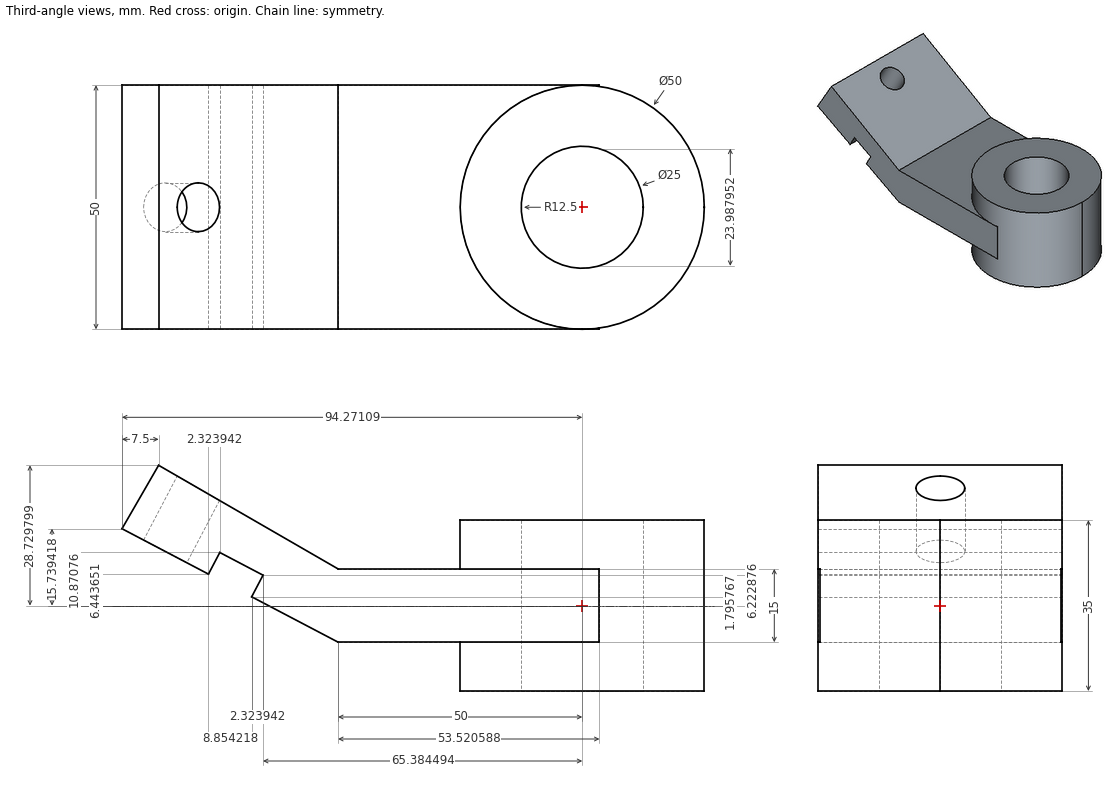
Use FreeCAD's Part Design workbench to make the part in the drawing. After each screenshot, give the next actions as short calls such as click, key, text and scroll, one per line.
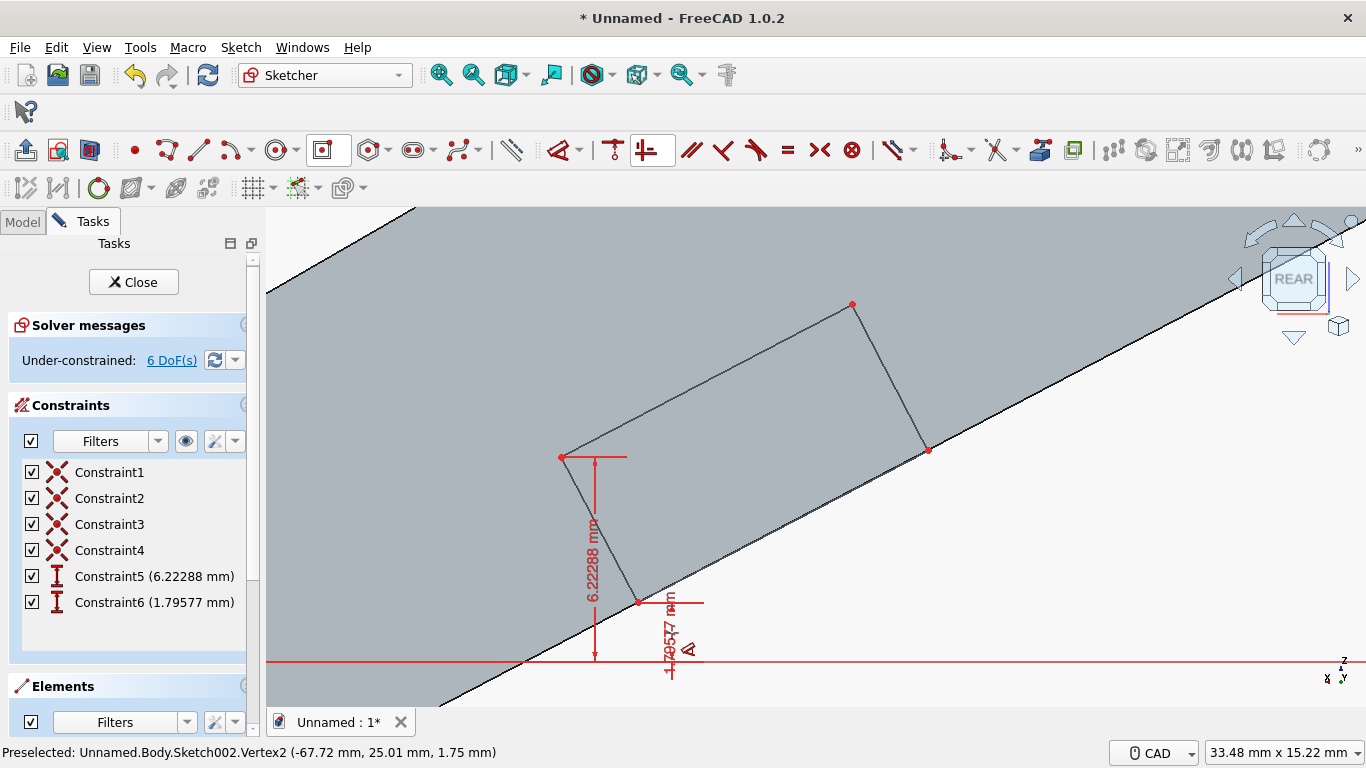
click(928, 451)
click(962, 556)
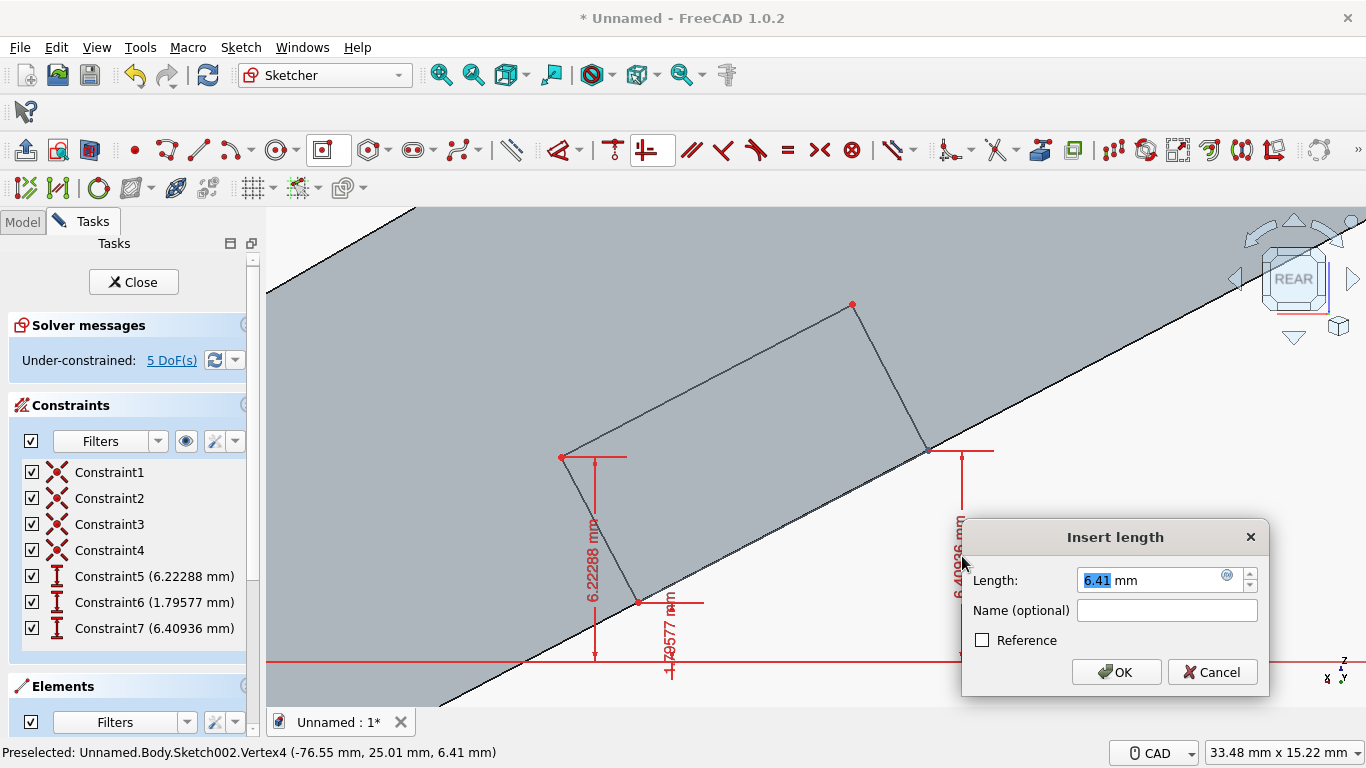
text(6.443651)
key(Return)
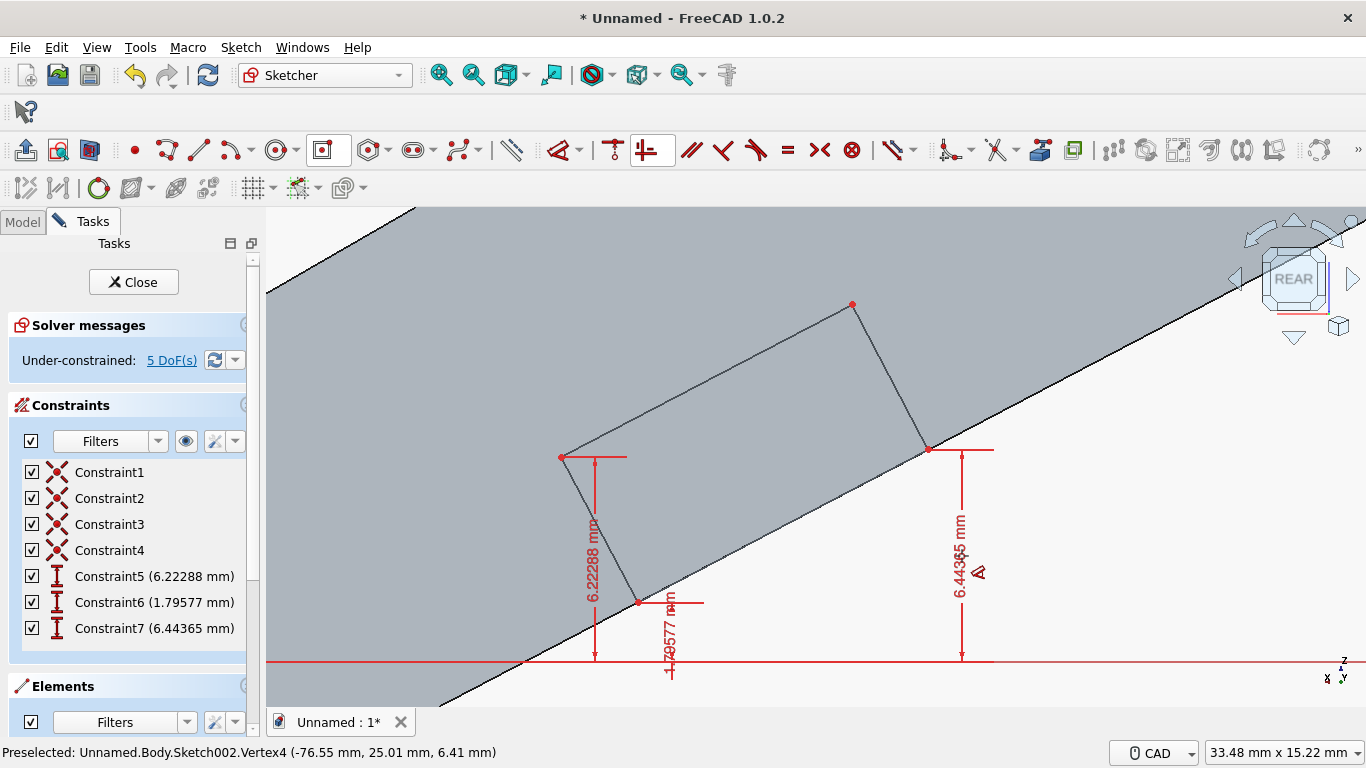
click(852, 305)
click(886, 401)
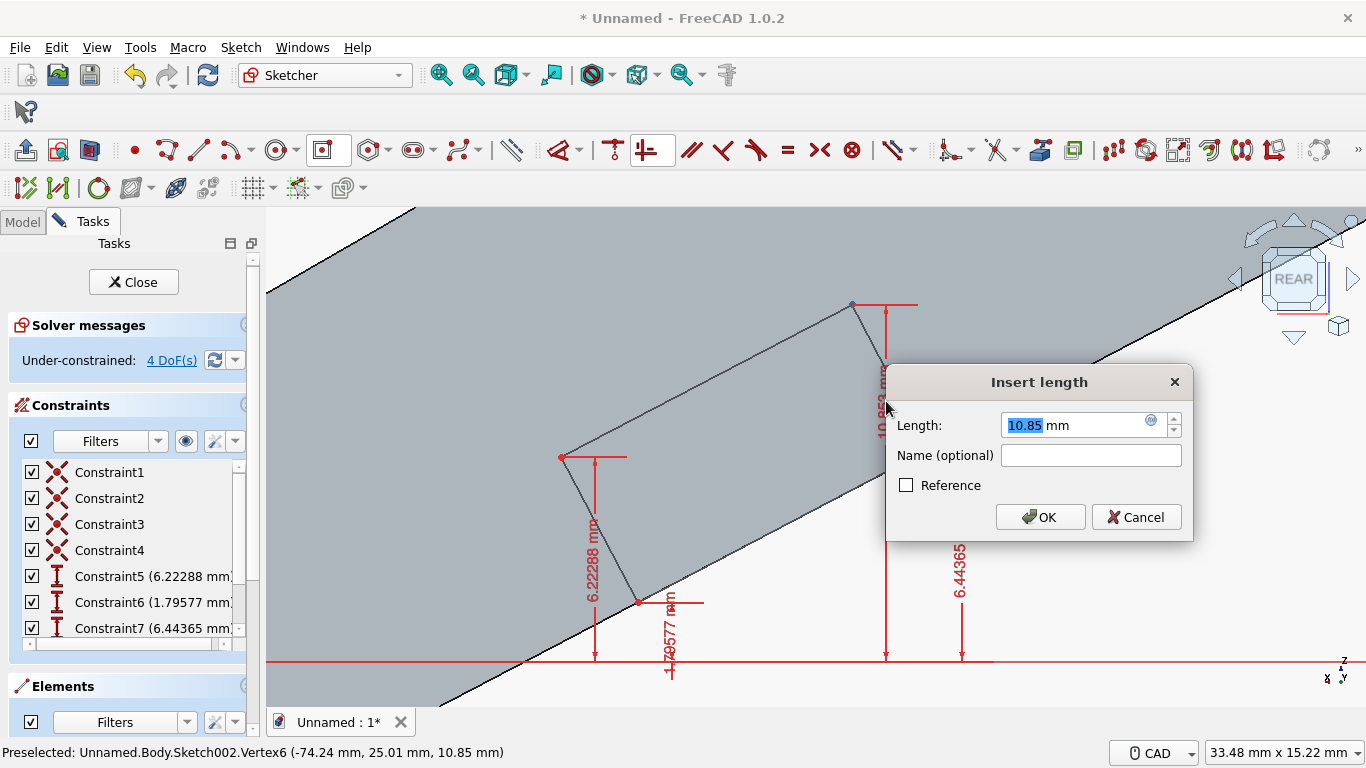
text(10.87076)
key(Return)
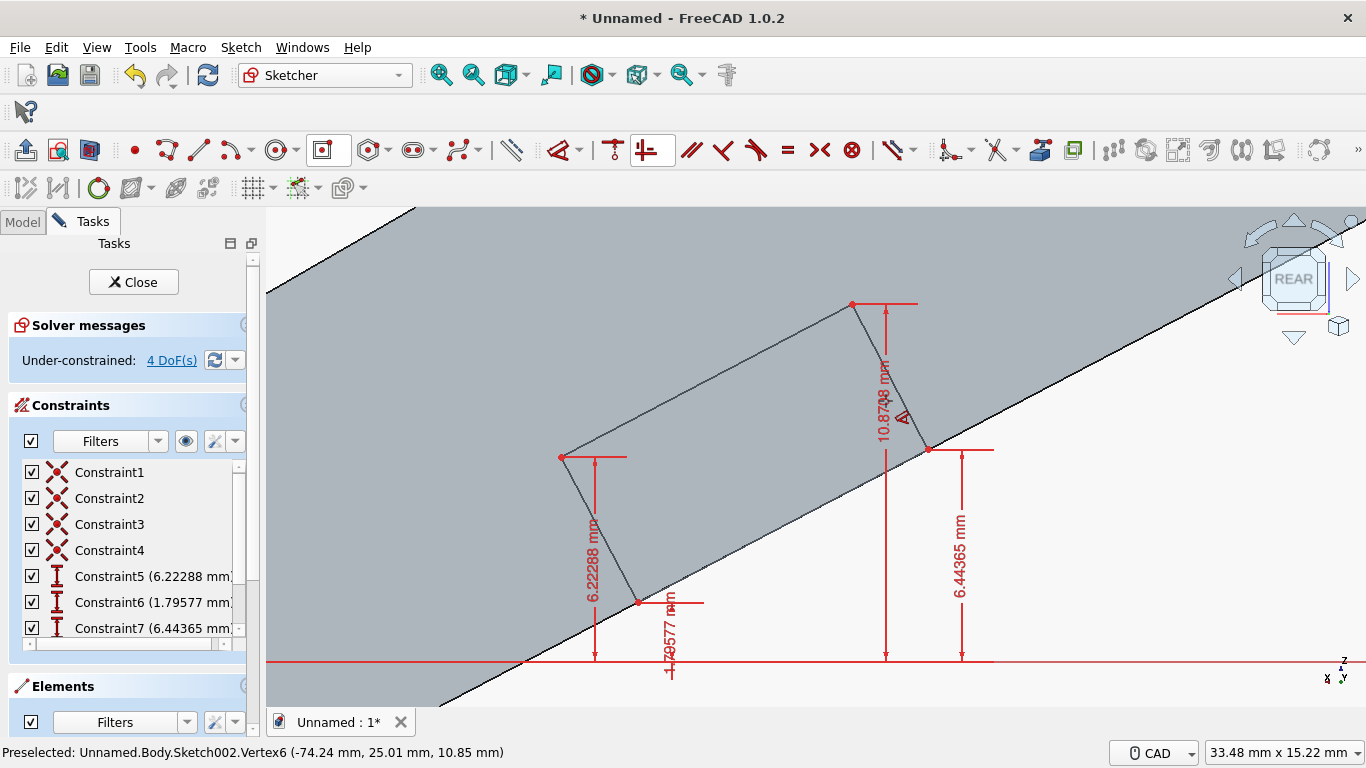
click(584, 501)
click(599, 637)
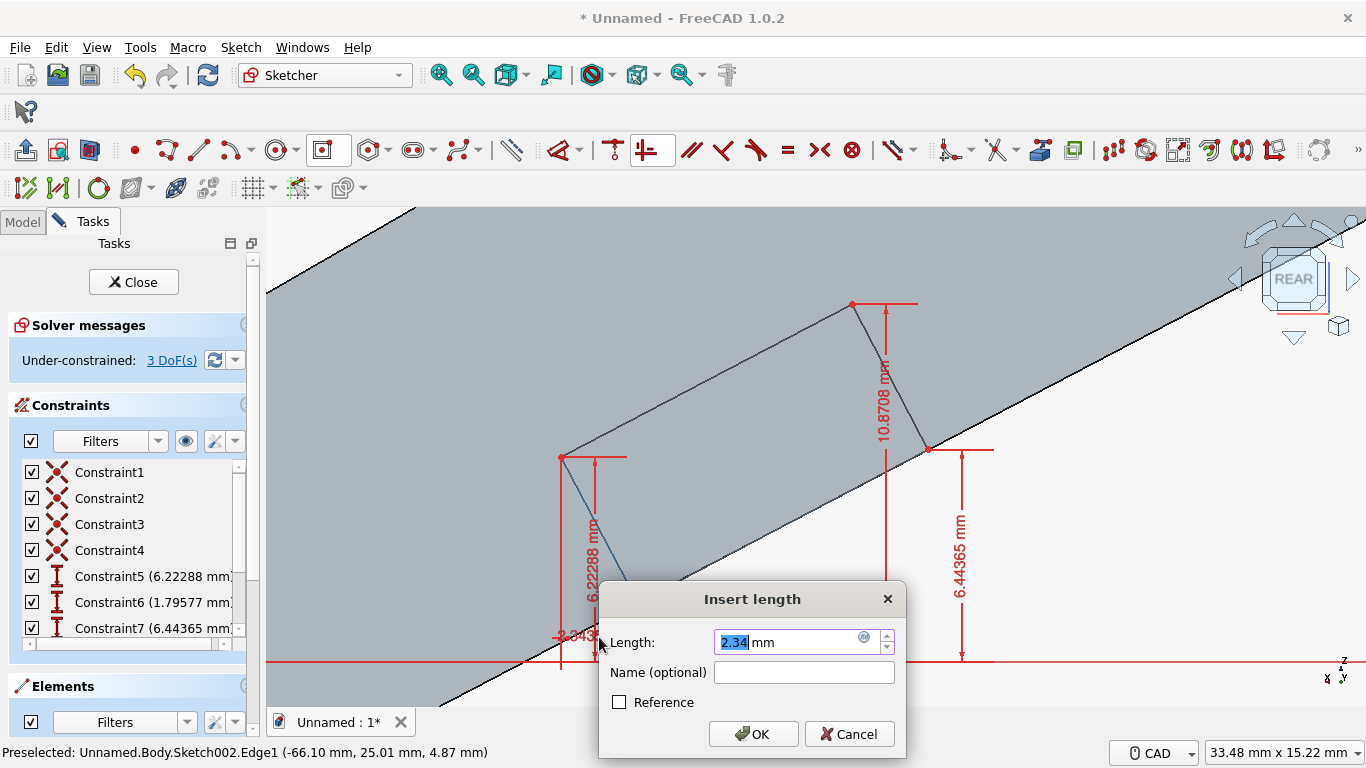
text(2.323942)
key(Return)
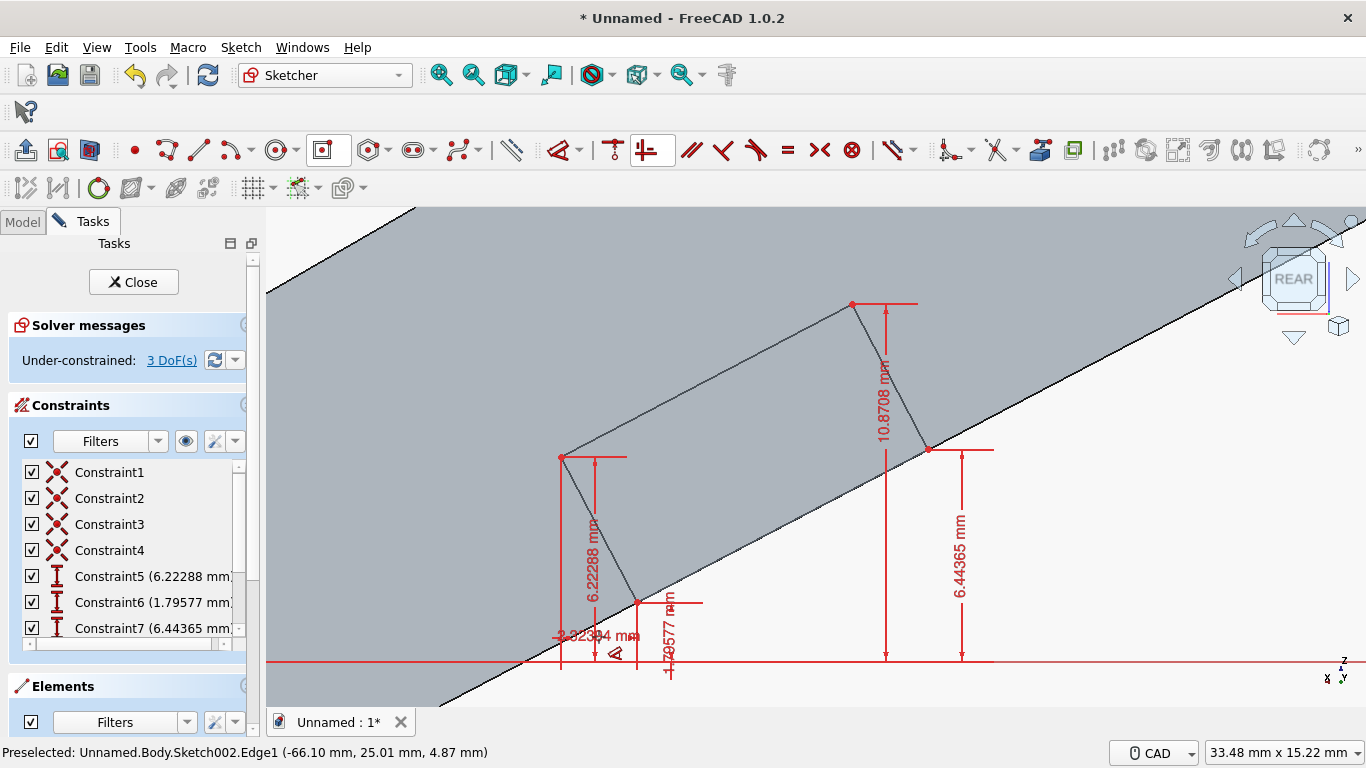
click(725, 557)
click(783, 637)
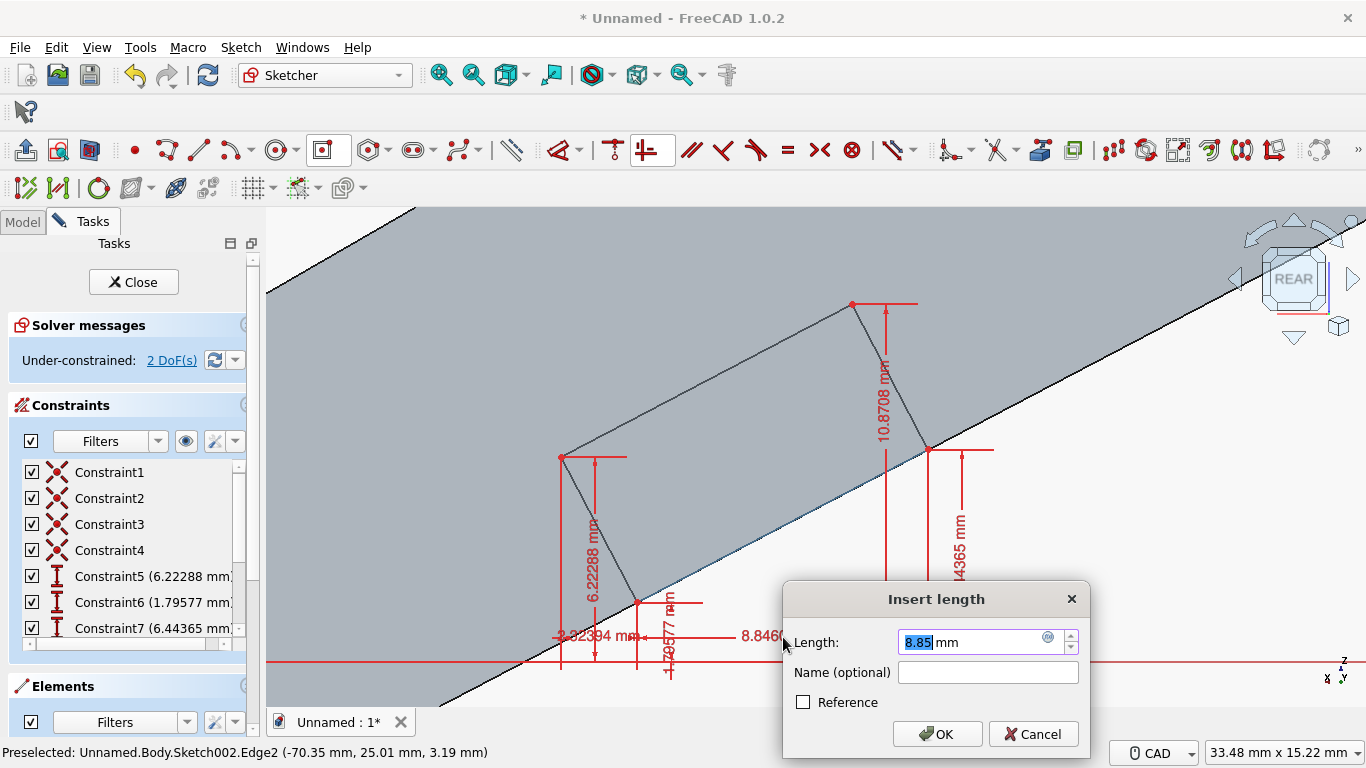
text(8.854218)
key(Return)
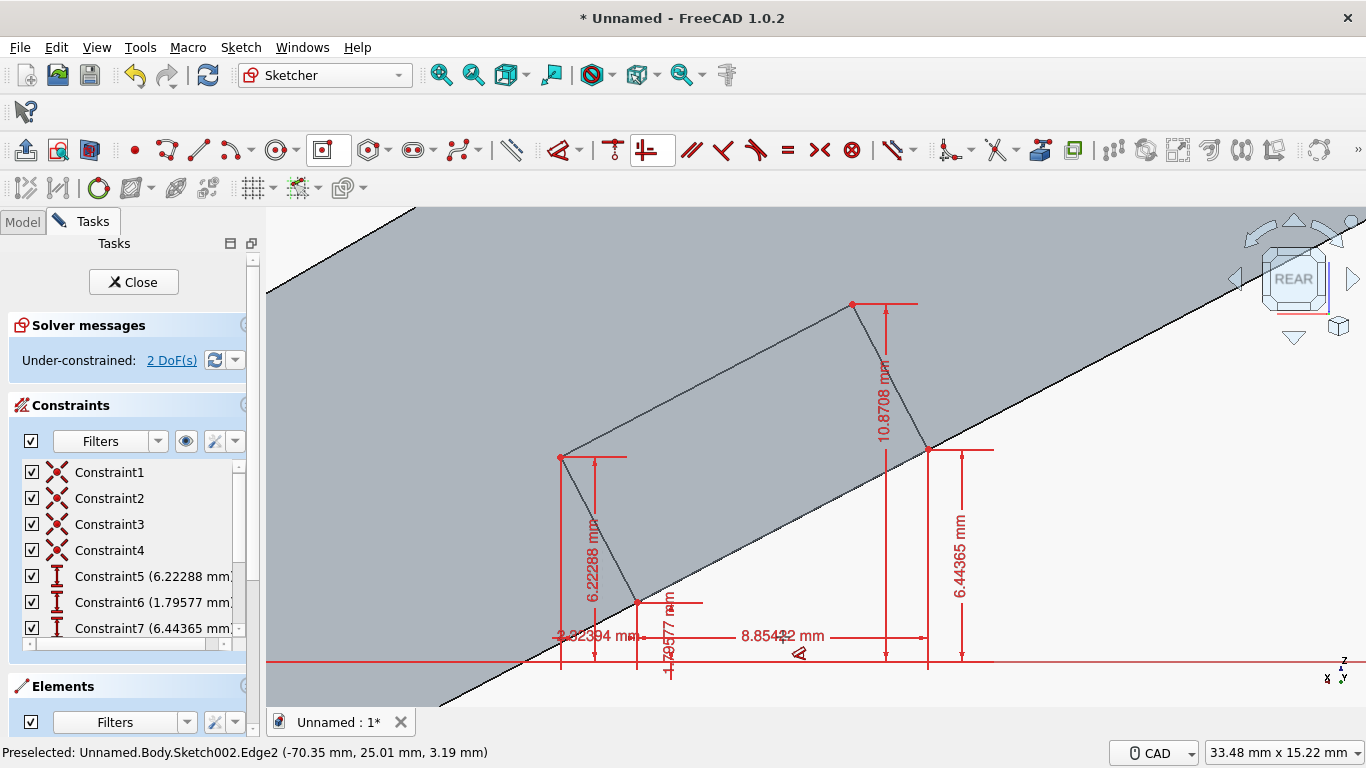
click(905, 406)
click(890, 270)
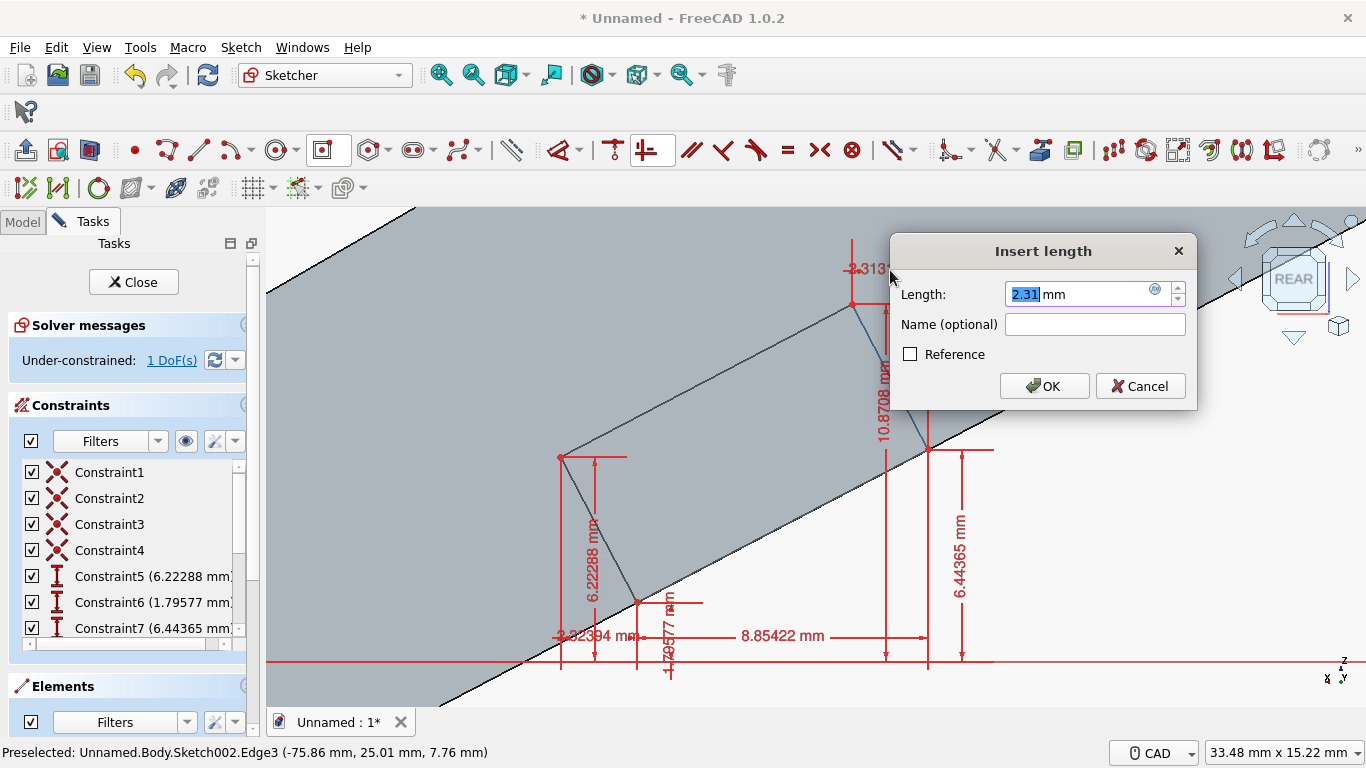
text(2.323942)
key(Return)